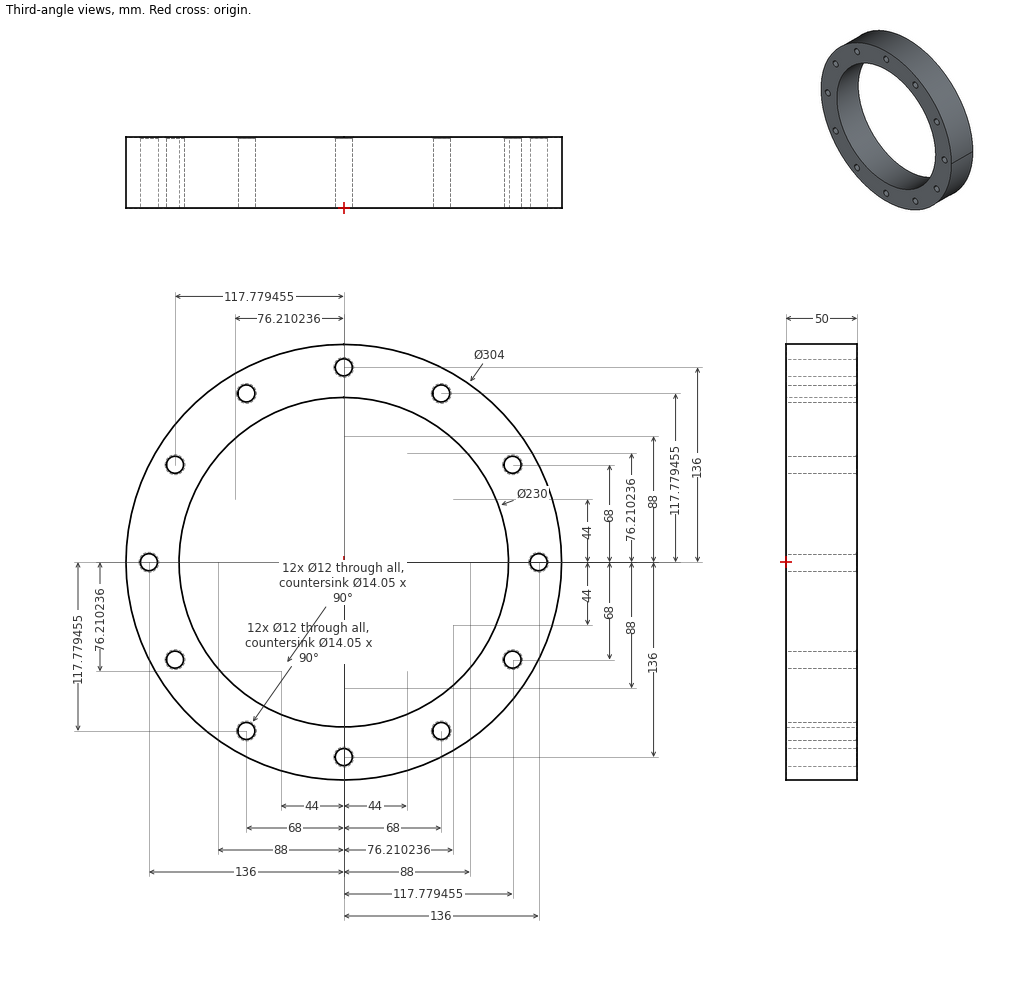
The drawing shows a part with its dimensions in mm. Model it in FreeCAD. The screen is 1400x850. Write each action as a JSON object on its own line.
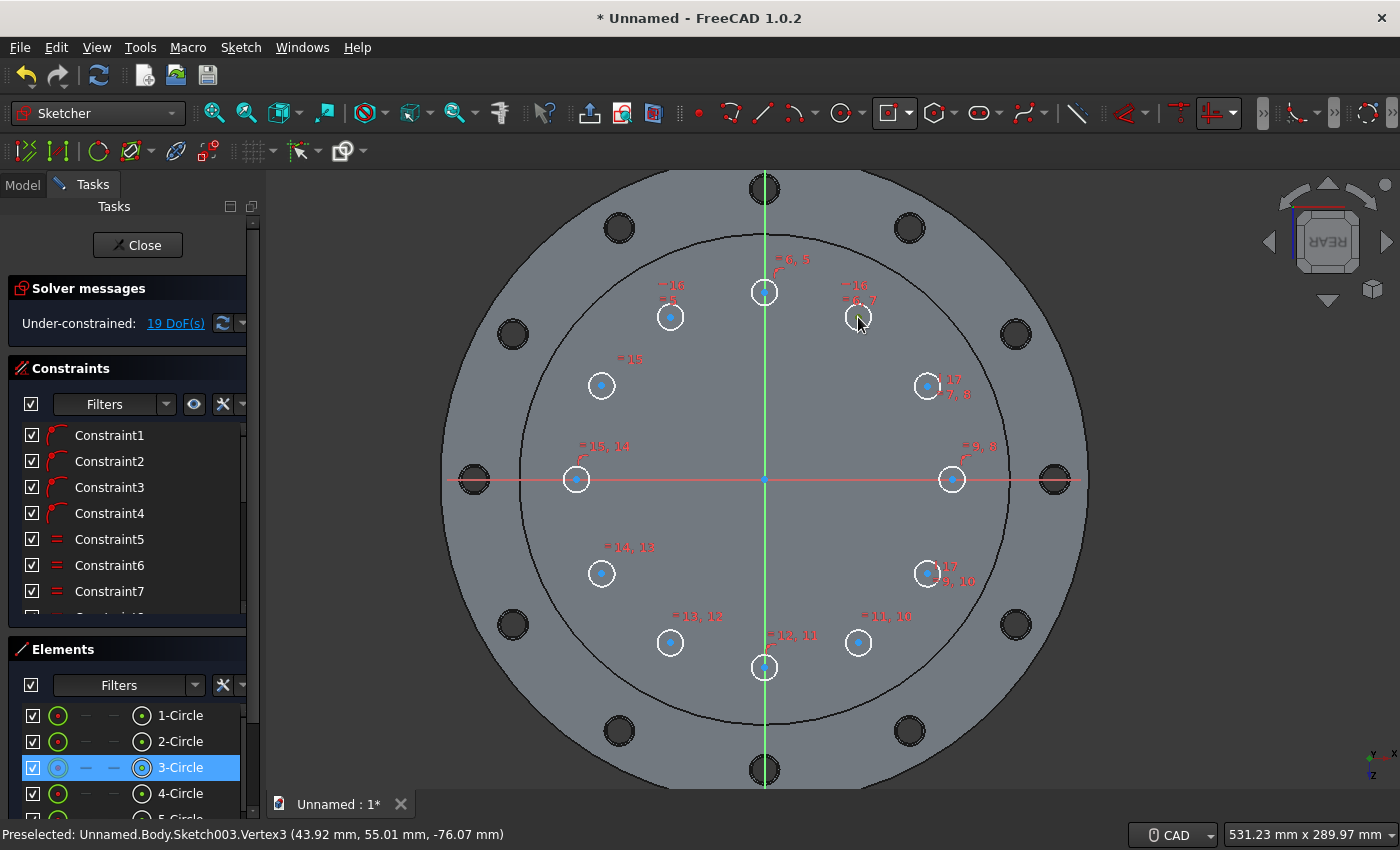
{"action": "left_click", "coordinate": [859, 643]}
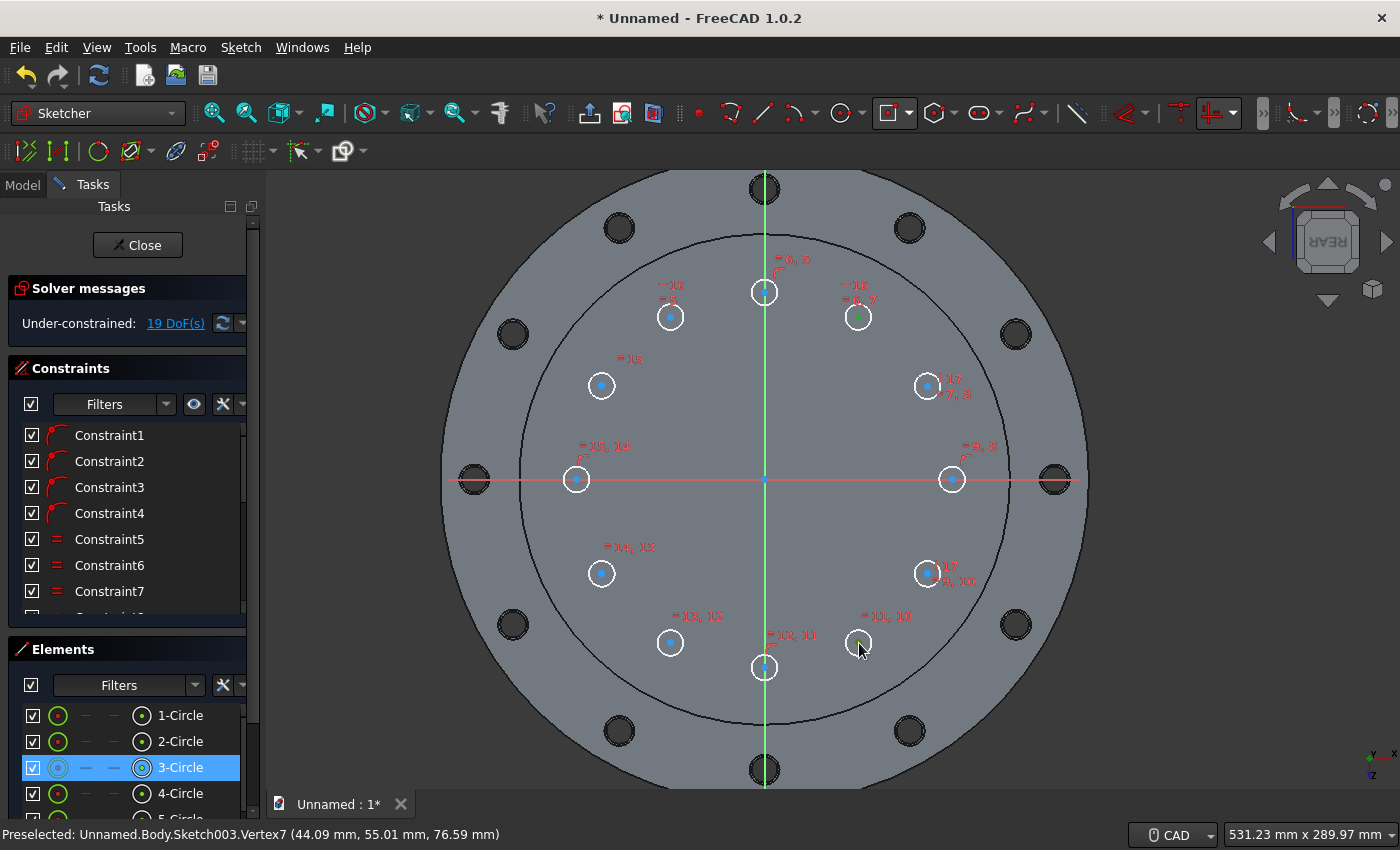
{"action": "left_click", "coordinate": [1236, 114]}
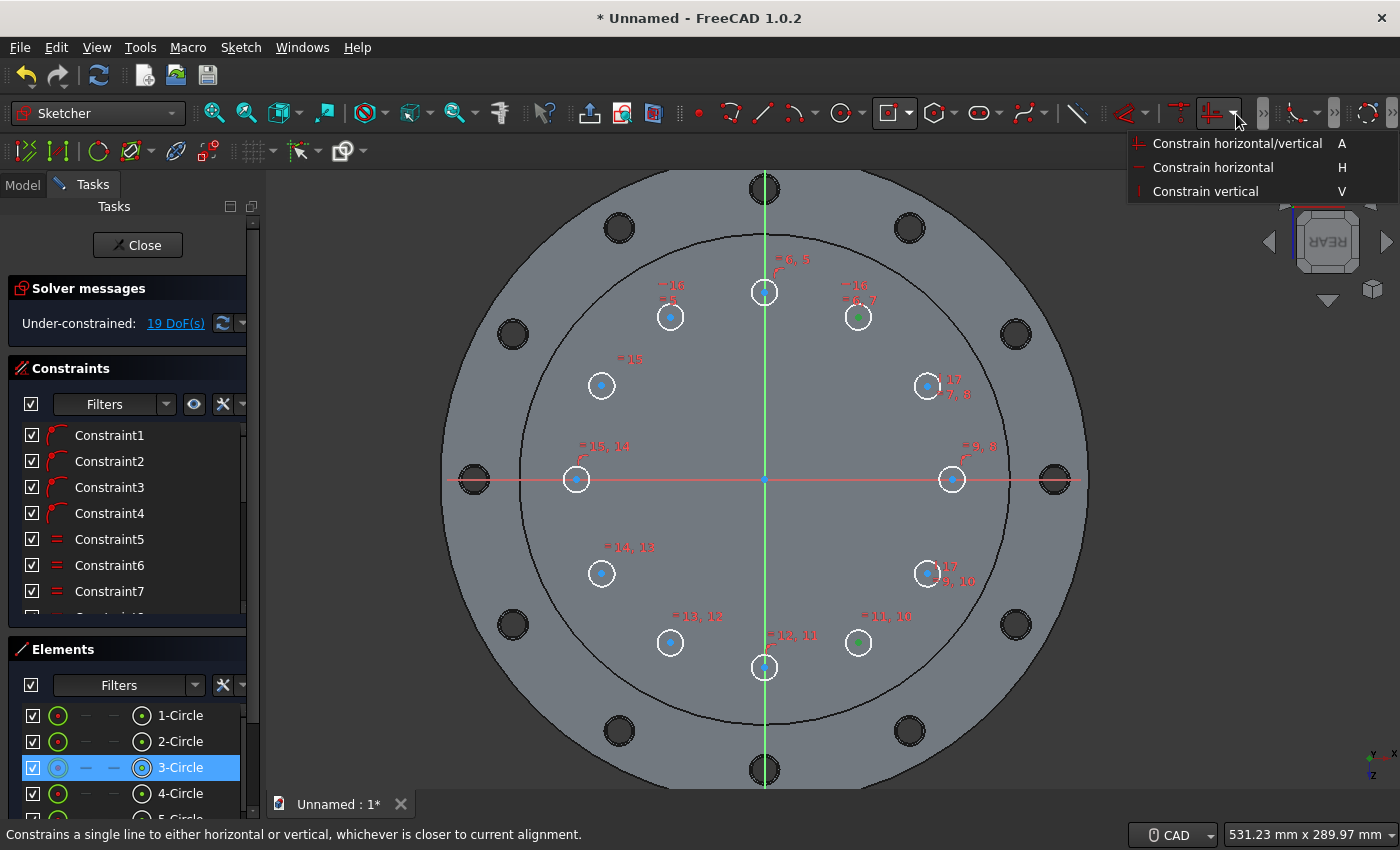
{"action": "left_click", "coordinate": [1263, 191]}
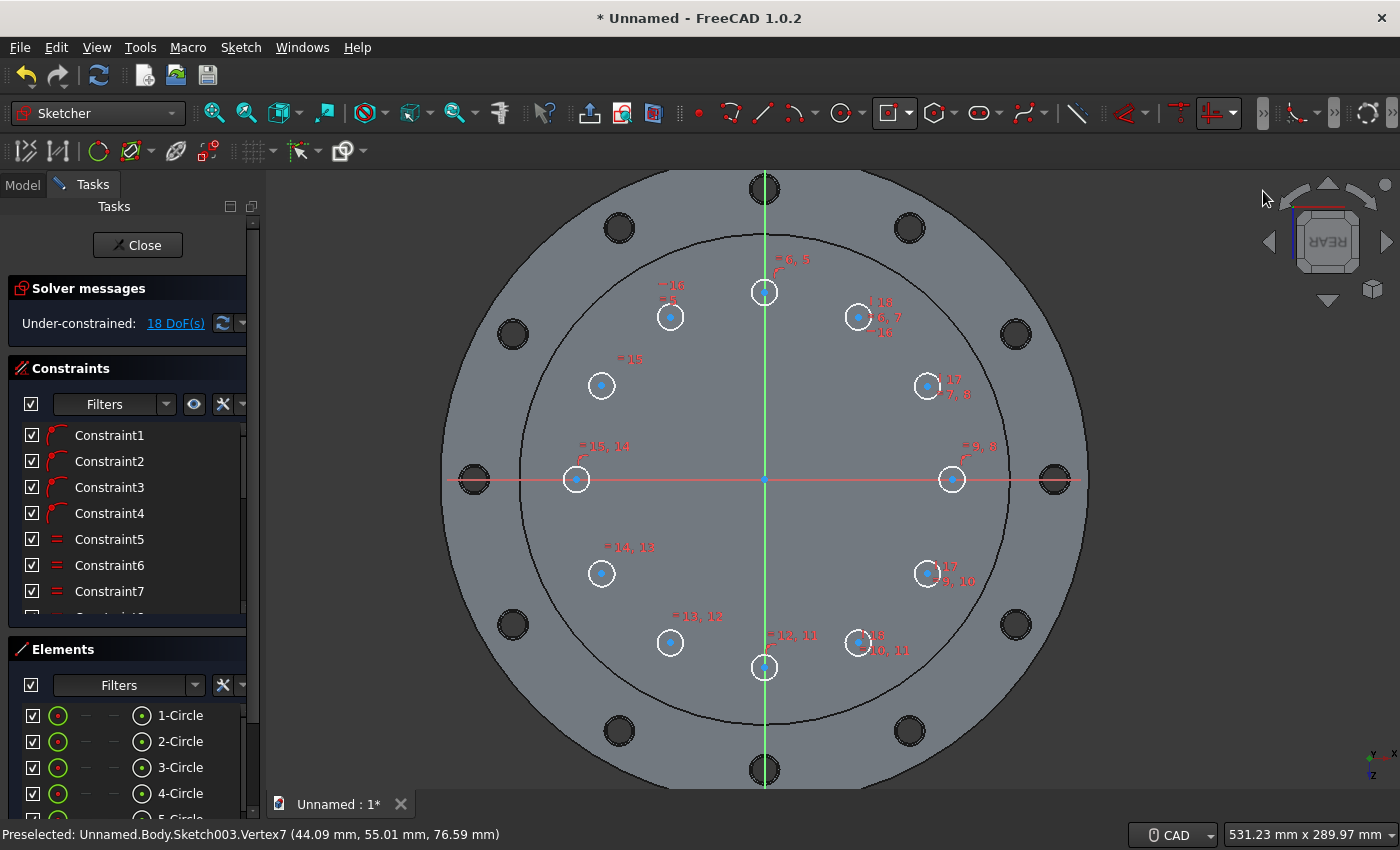
{"action": "left_click", "coordinate": [671, 317]}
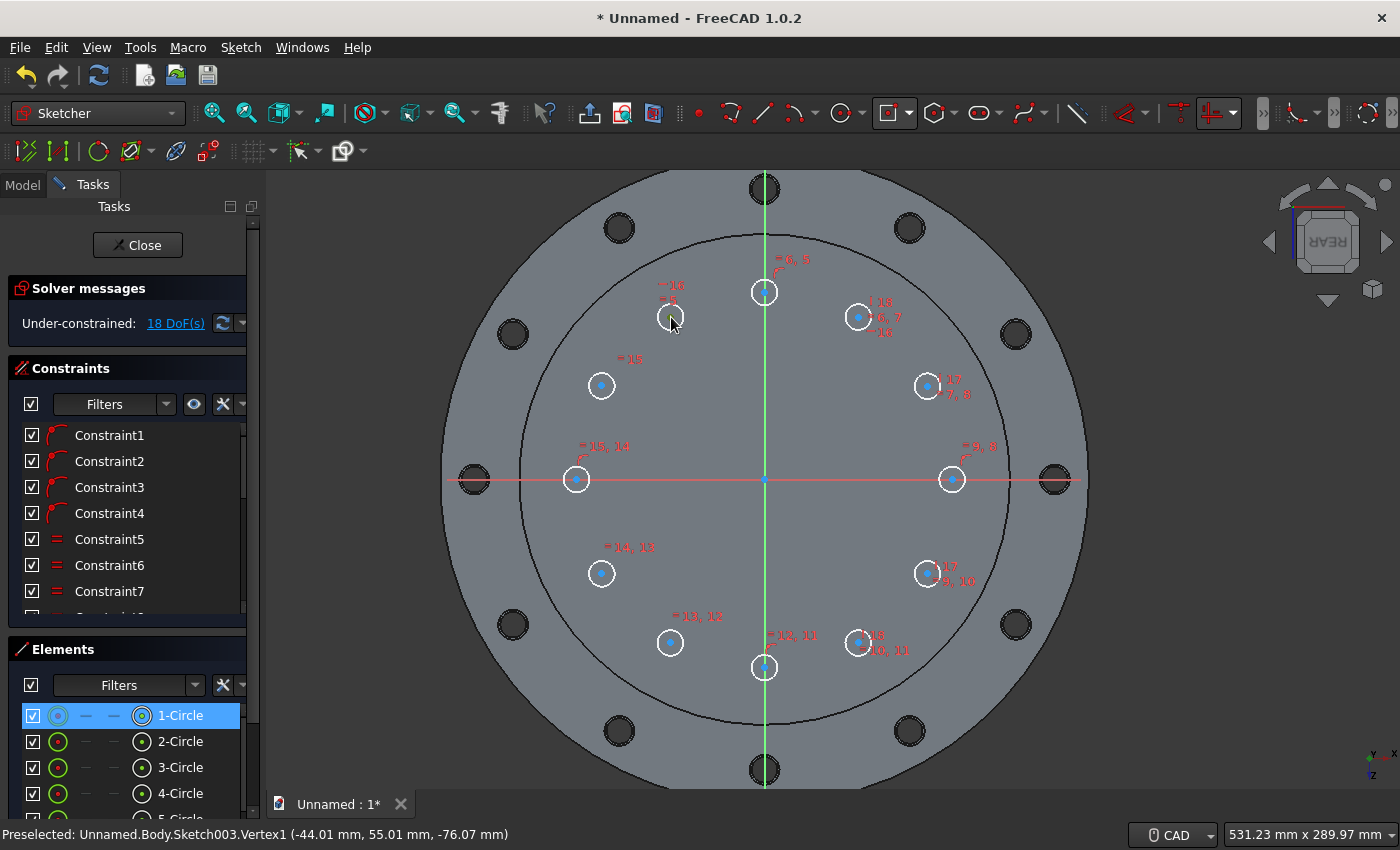
{"action": "left_click", "coordinate": [670, 643]}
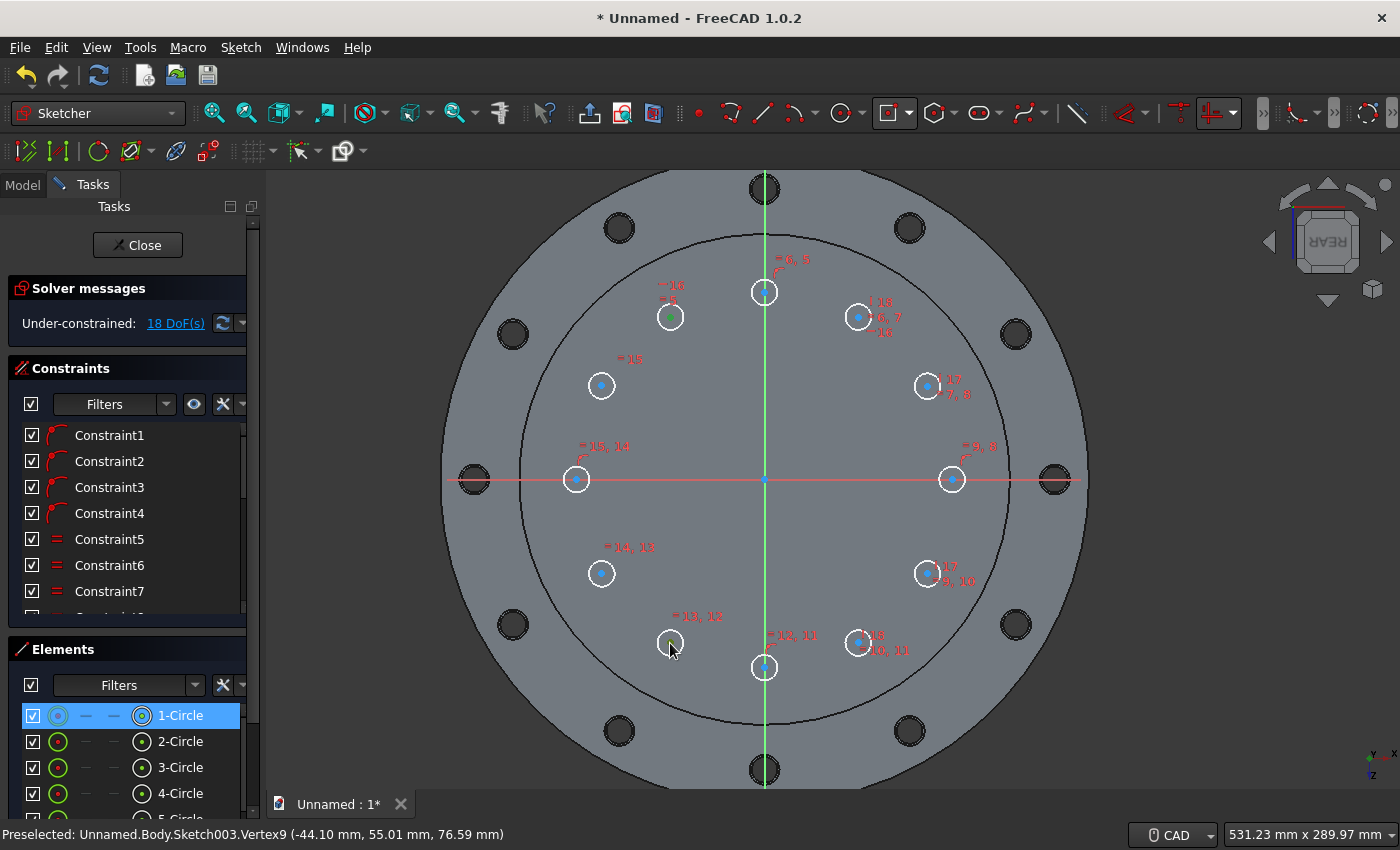
{"action": "left_click", "coordinate": [1236, 114]}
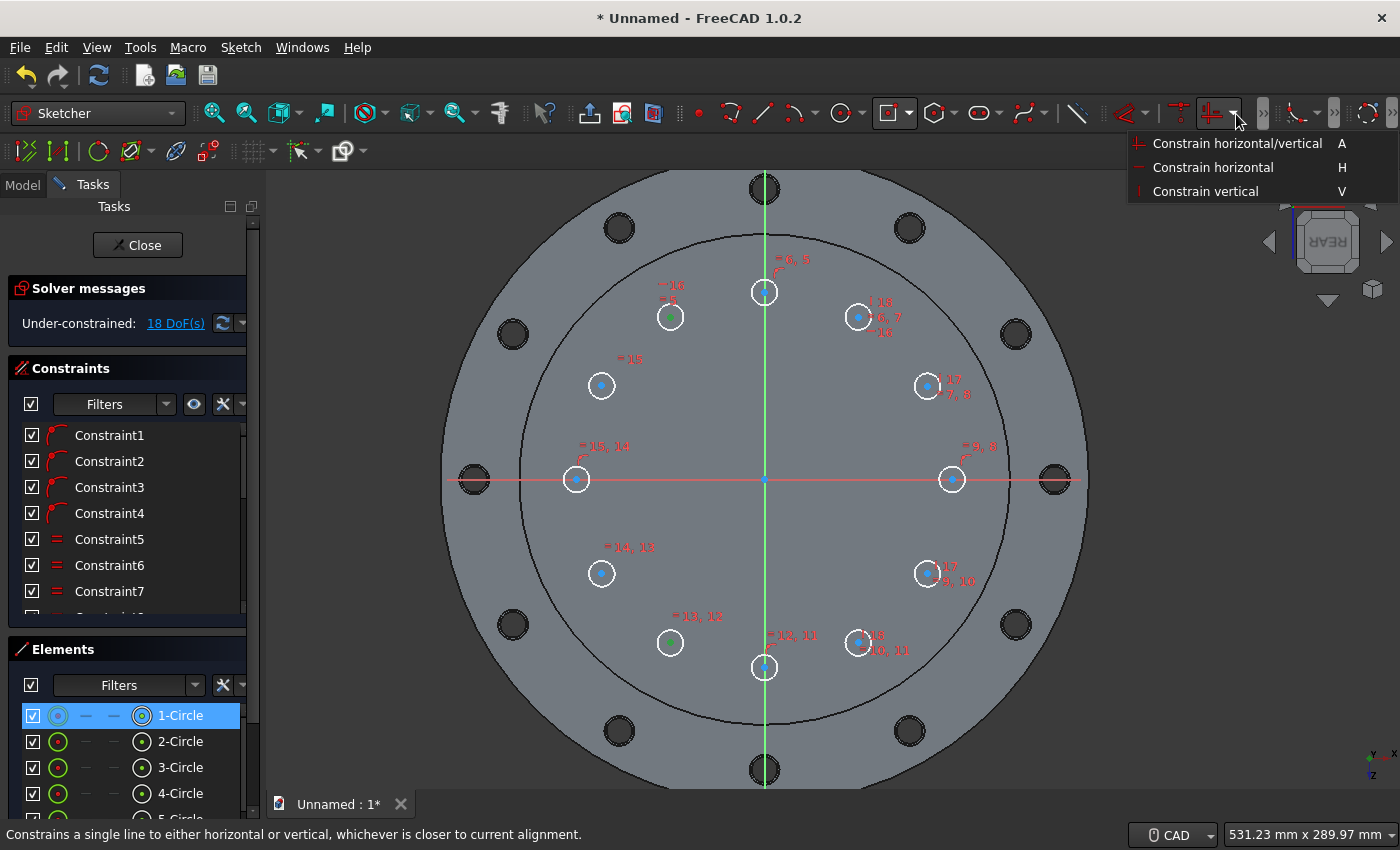
{"action": "left_click", "coordinate": [1263, 191]}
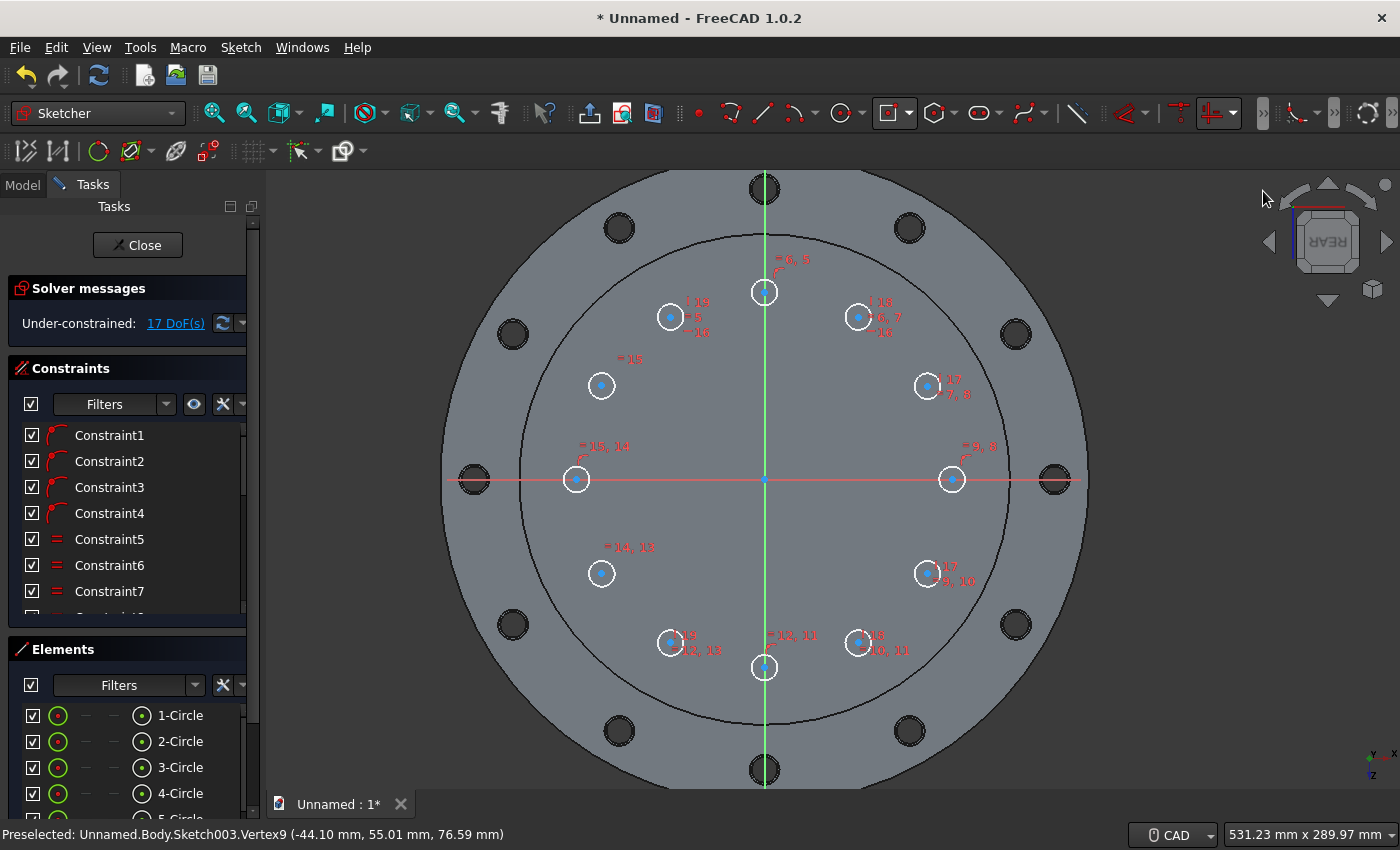
{"action": "left_click", "coordinate": [856, 645]}